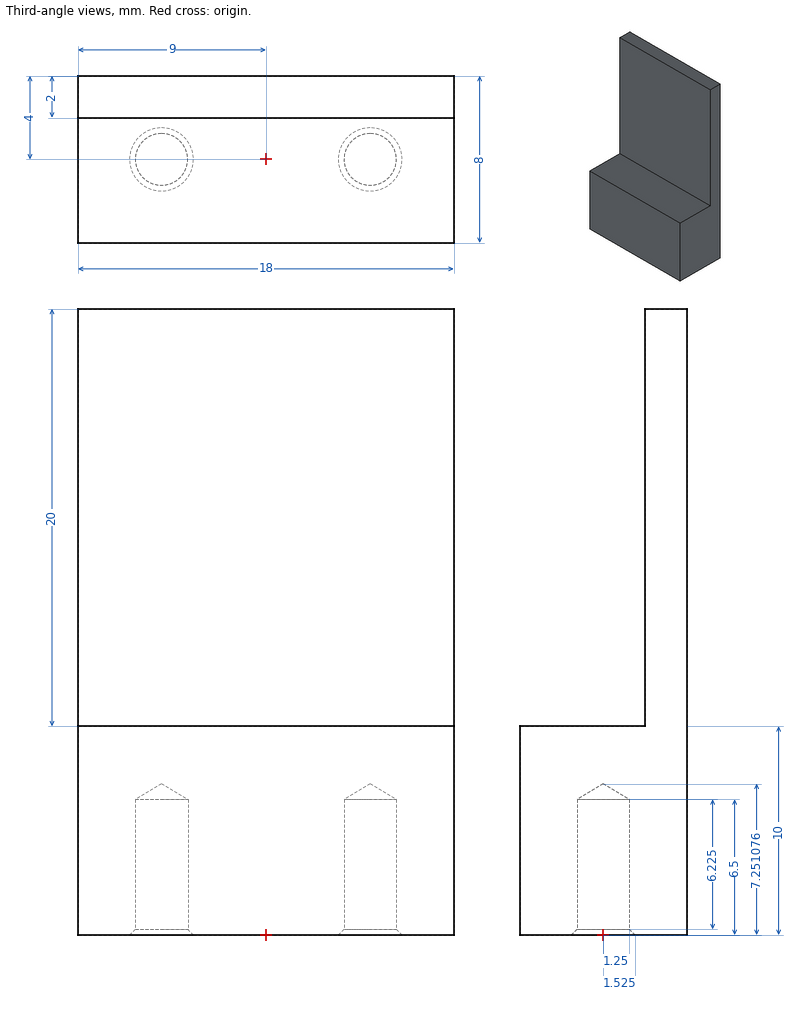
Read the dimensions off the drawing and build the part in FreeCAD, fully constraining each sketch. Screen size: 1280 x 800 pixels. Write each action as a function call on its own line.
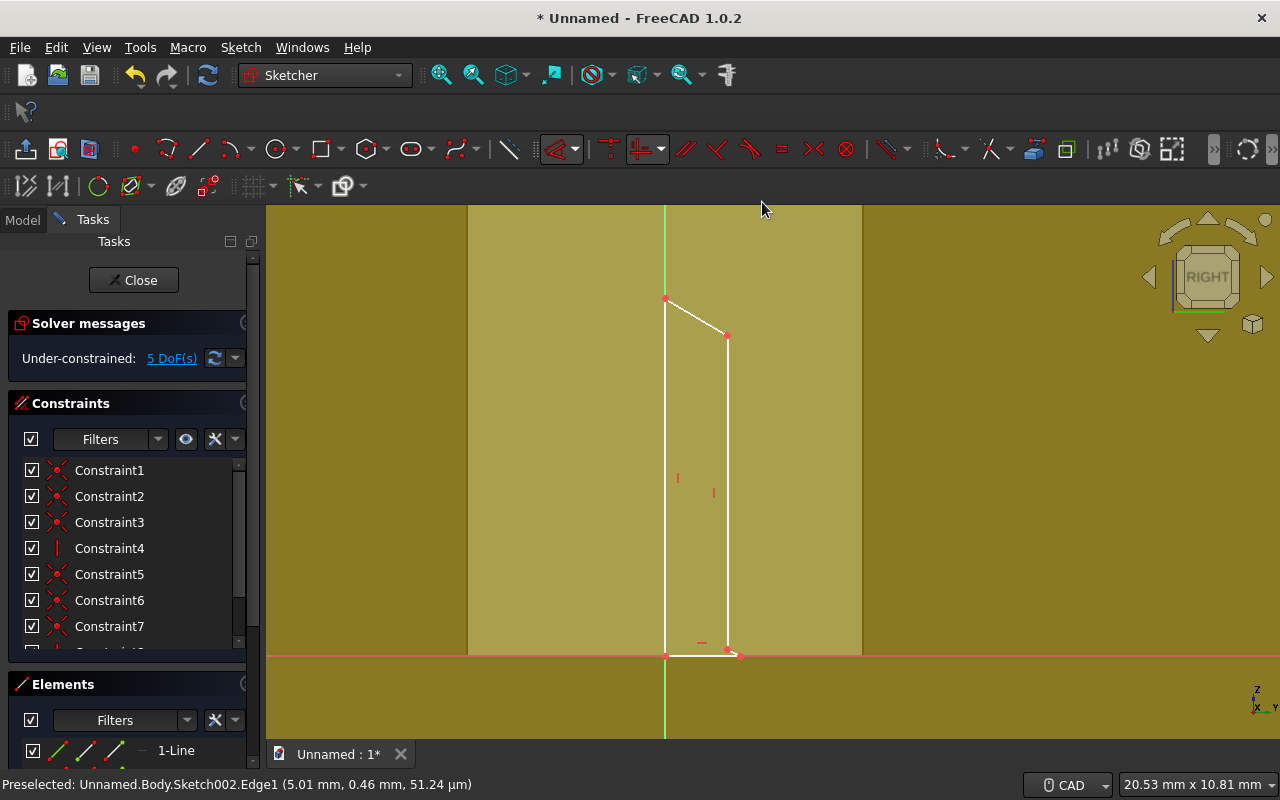
click(728, 336)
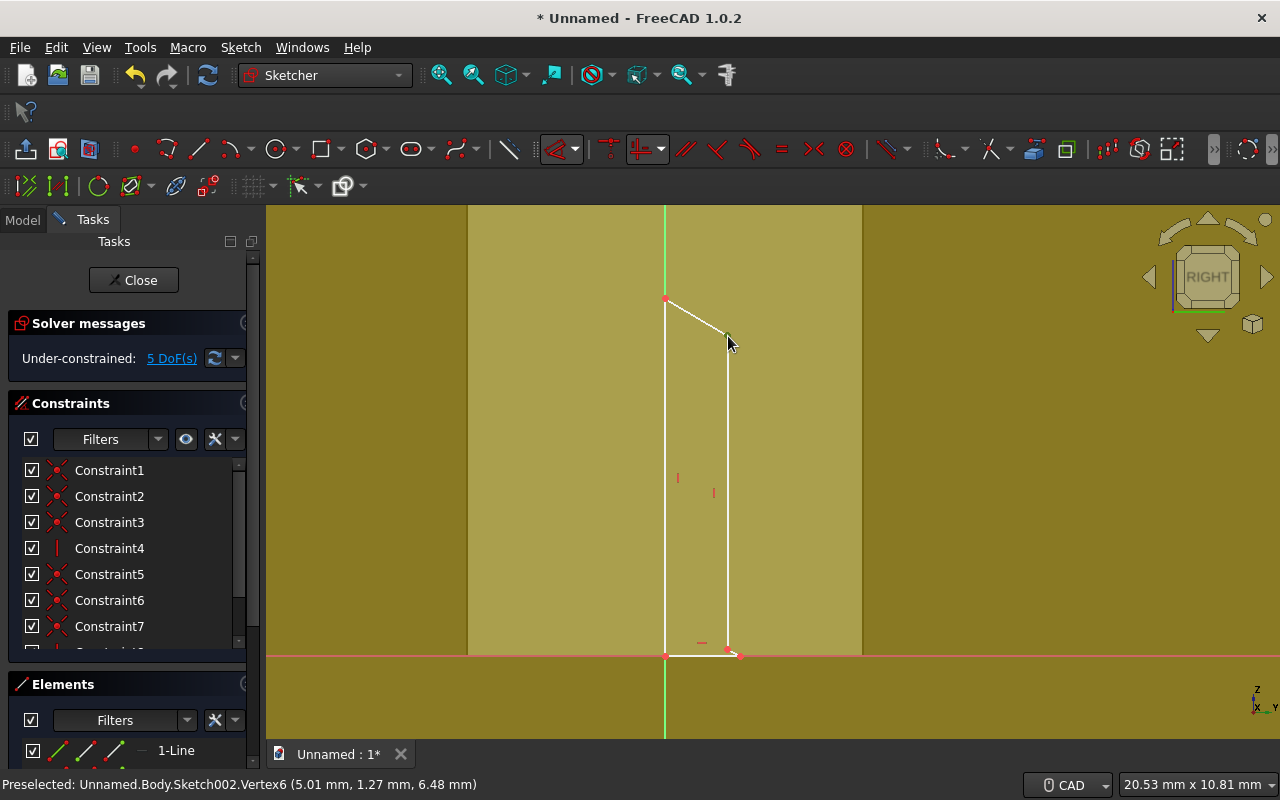
click(578, 150)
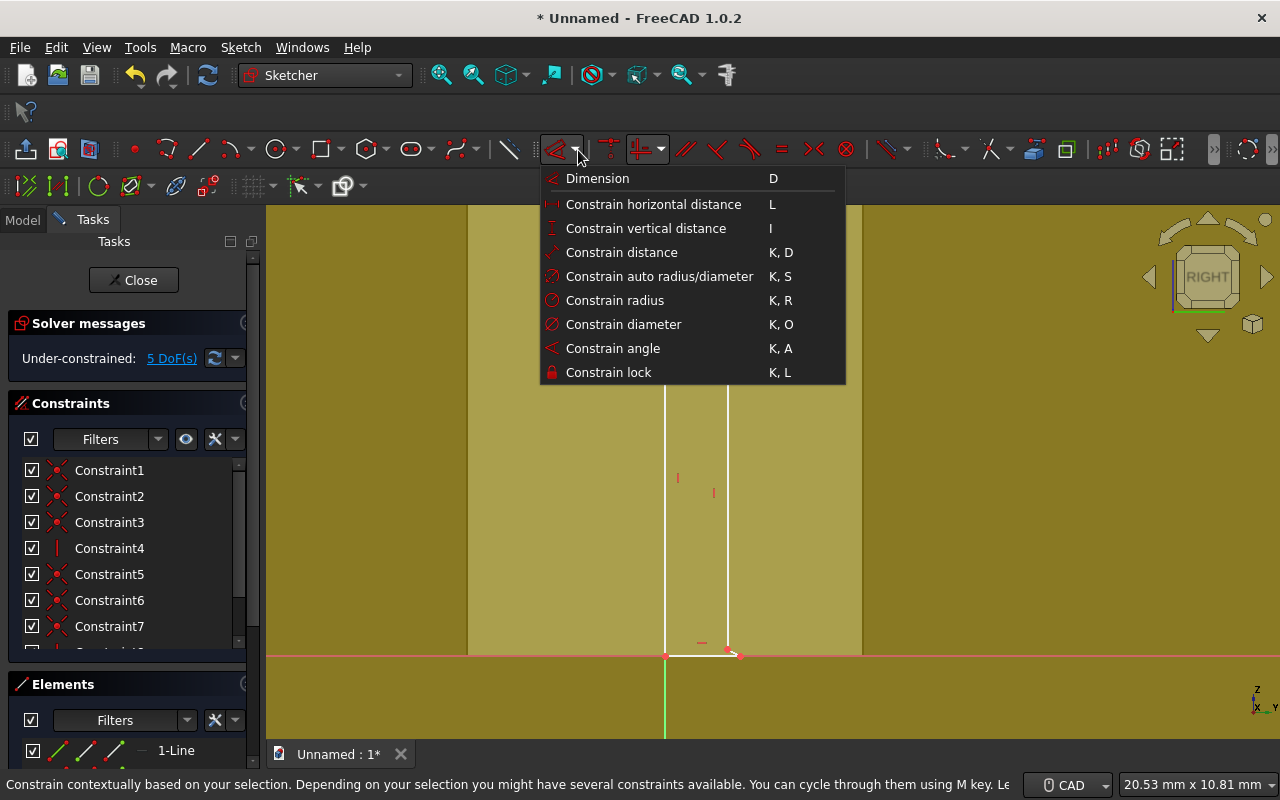
click(693, 228)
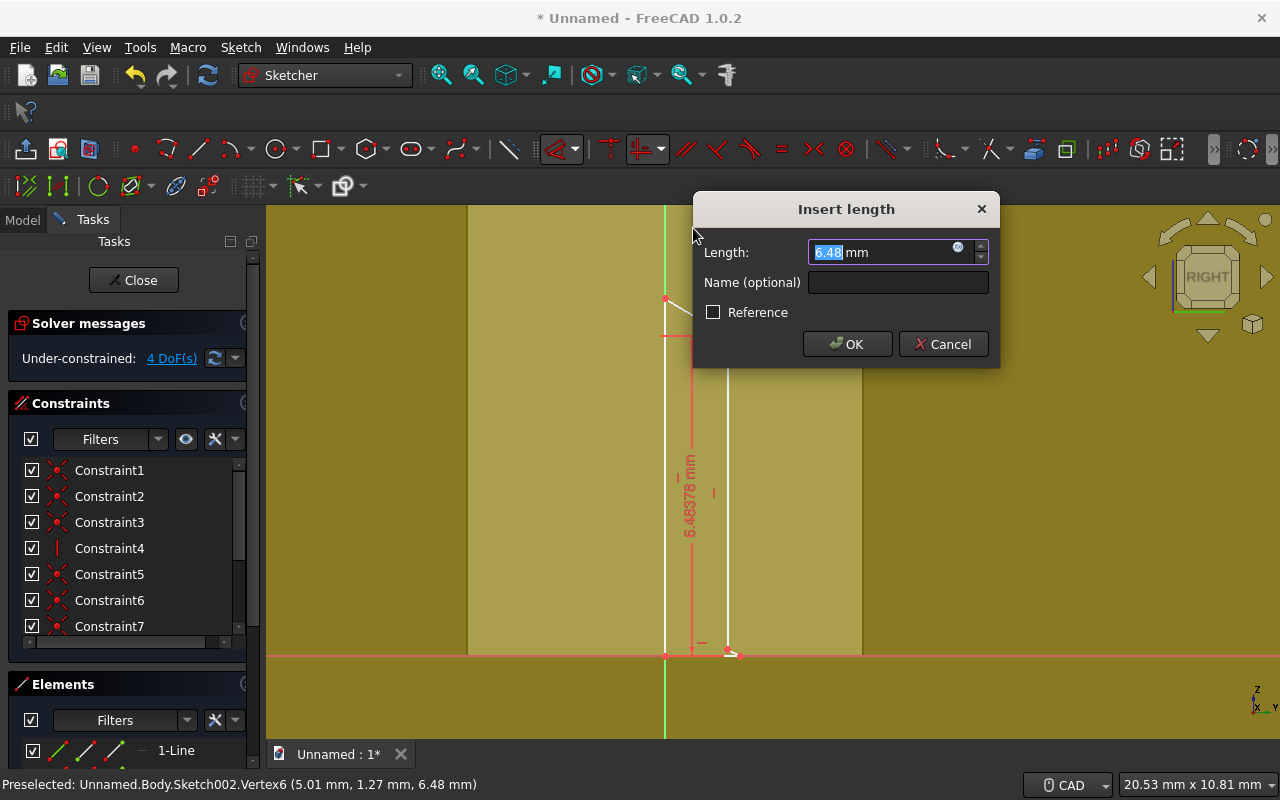
text(6.5)
key(Return)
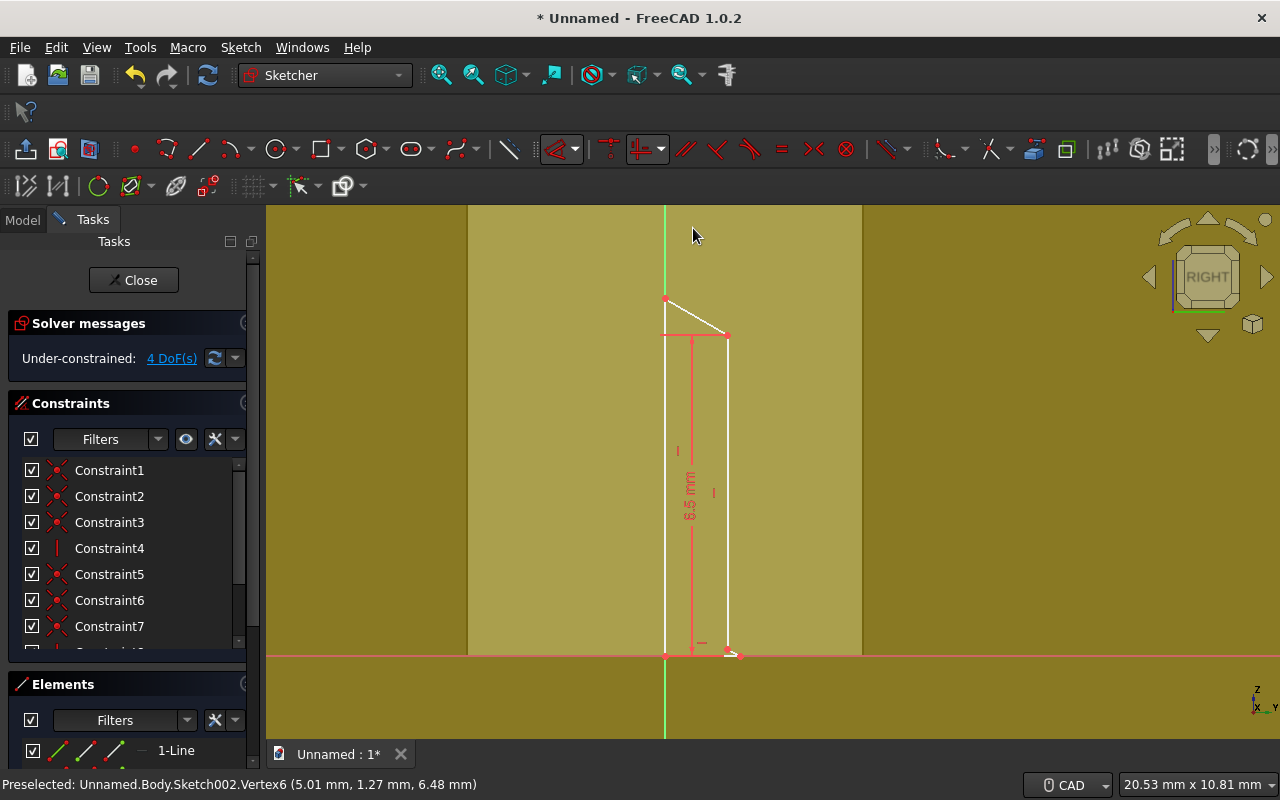
click(688, 656)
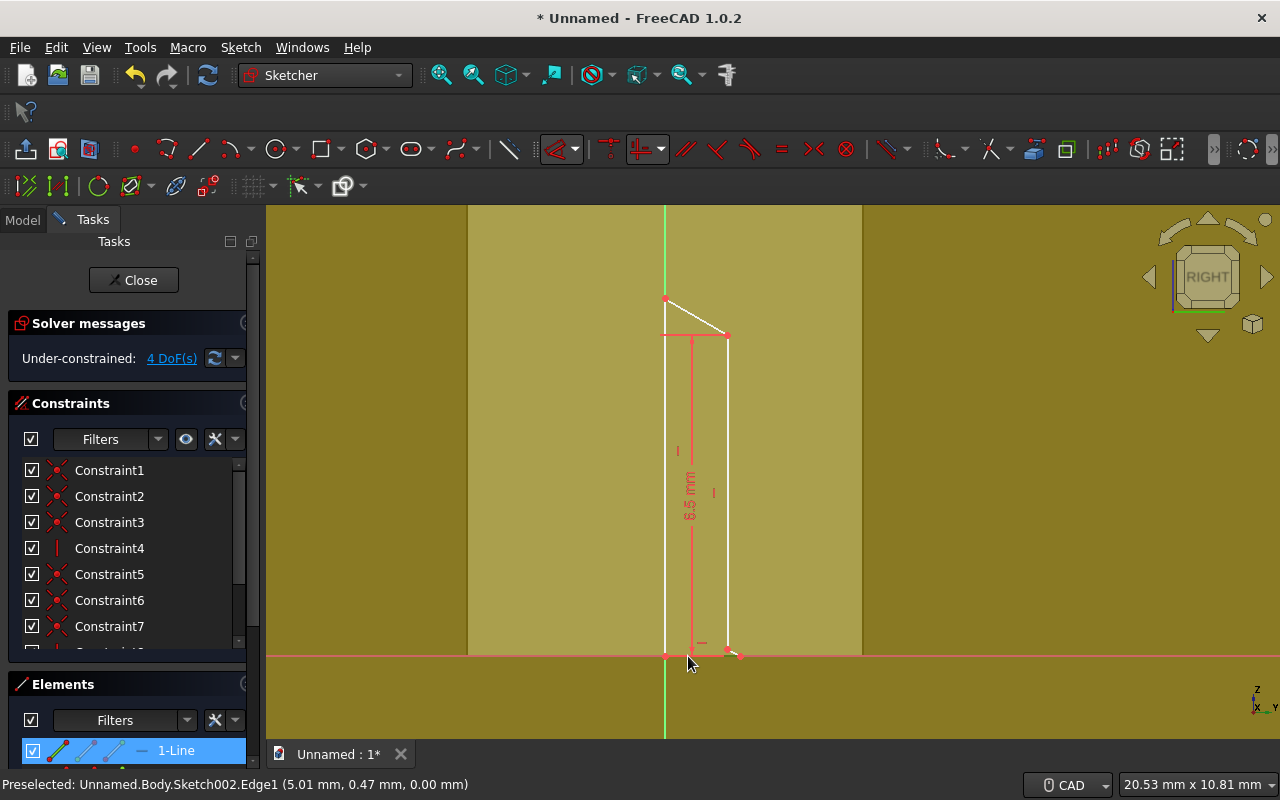
click(578, 150)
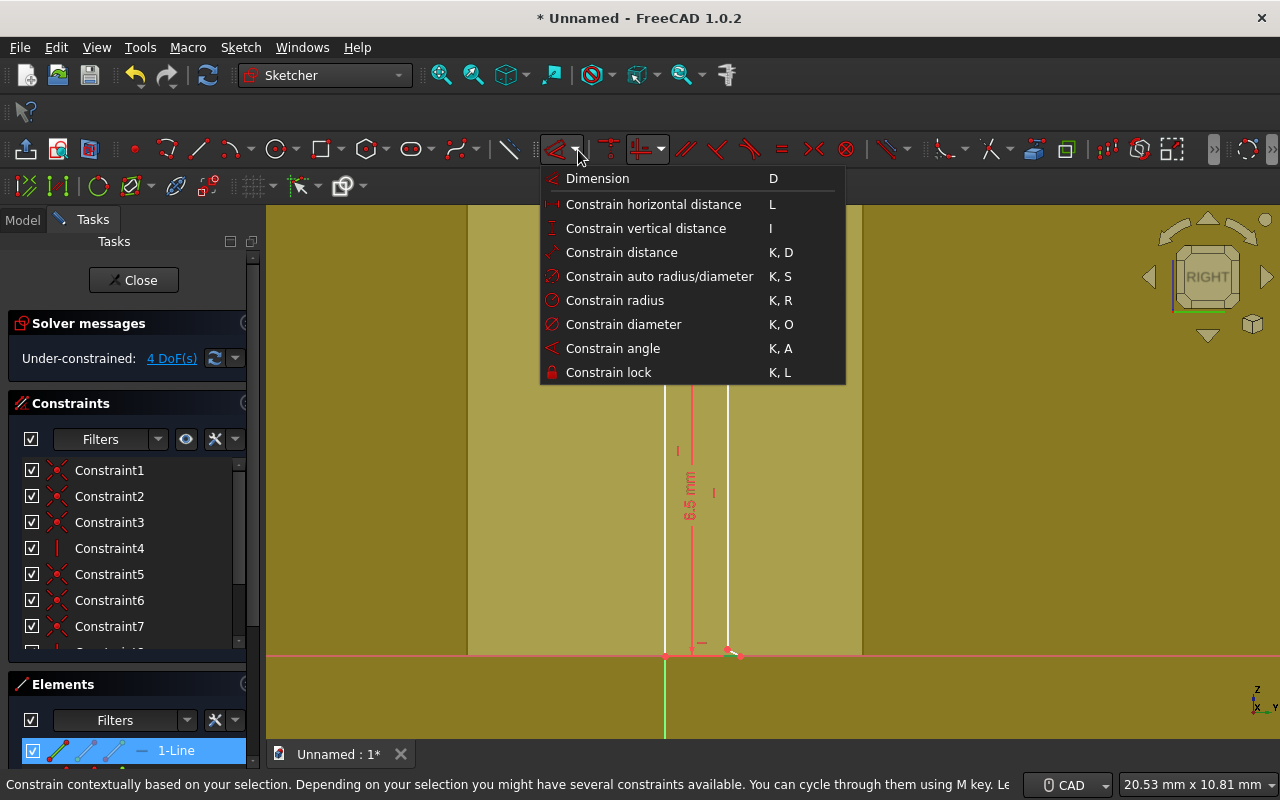
click(693, 204)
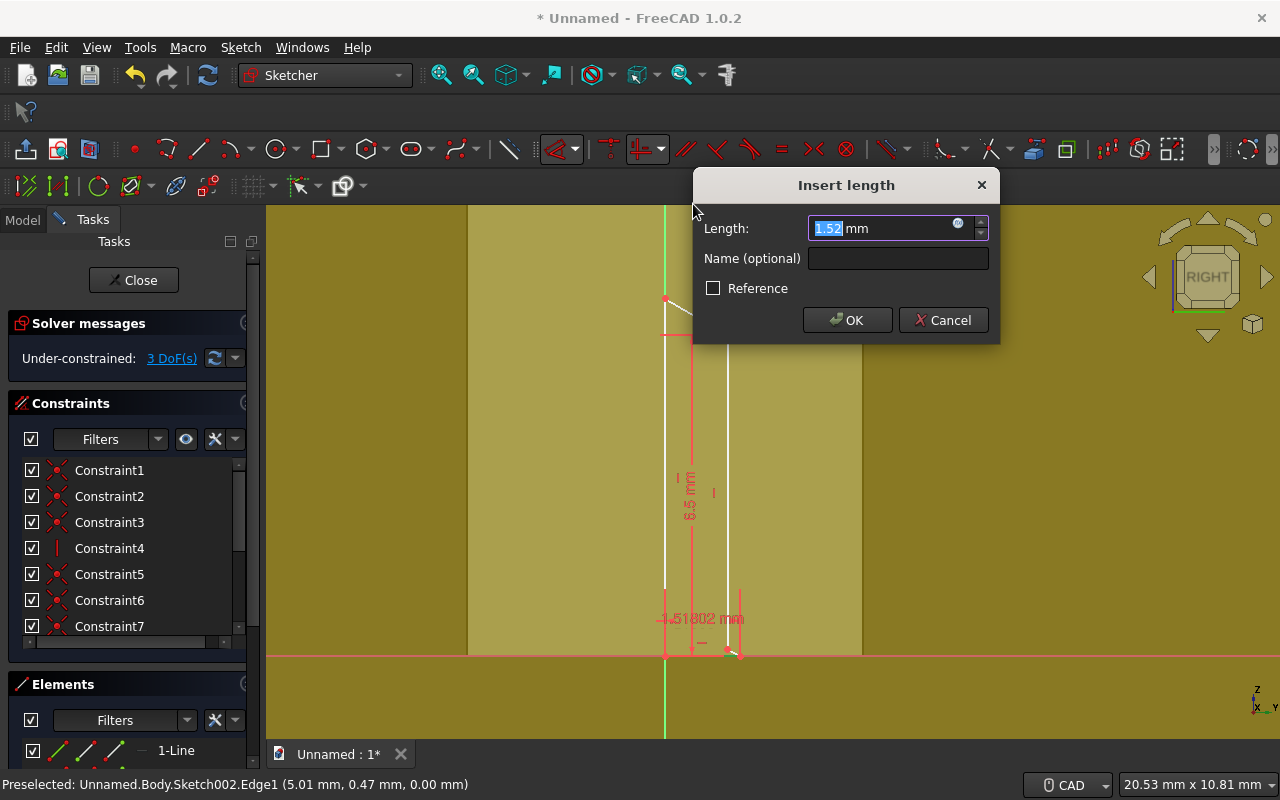
text(1.525)
key(Return)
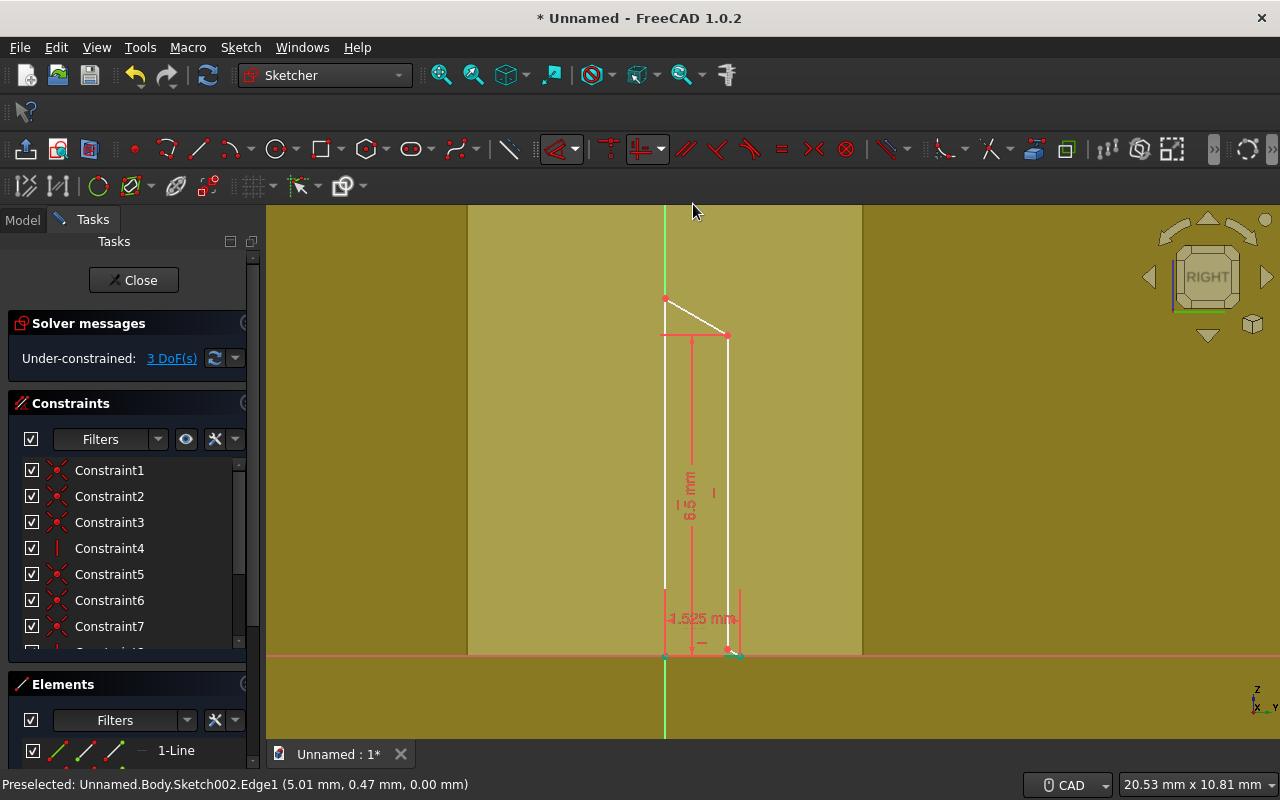
click(728, 555)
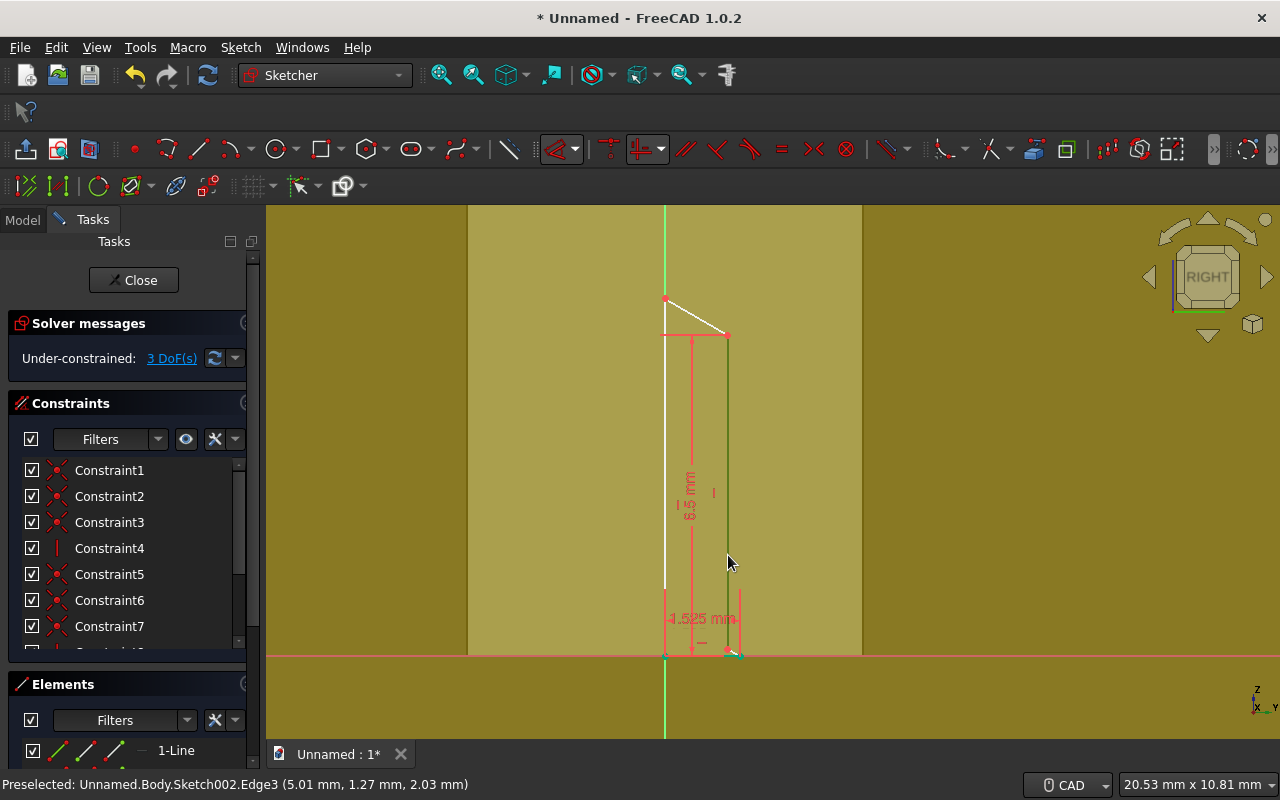
click(578, 150)